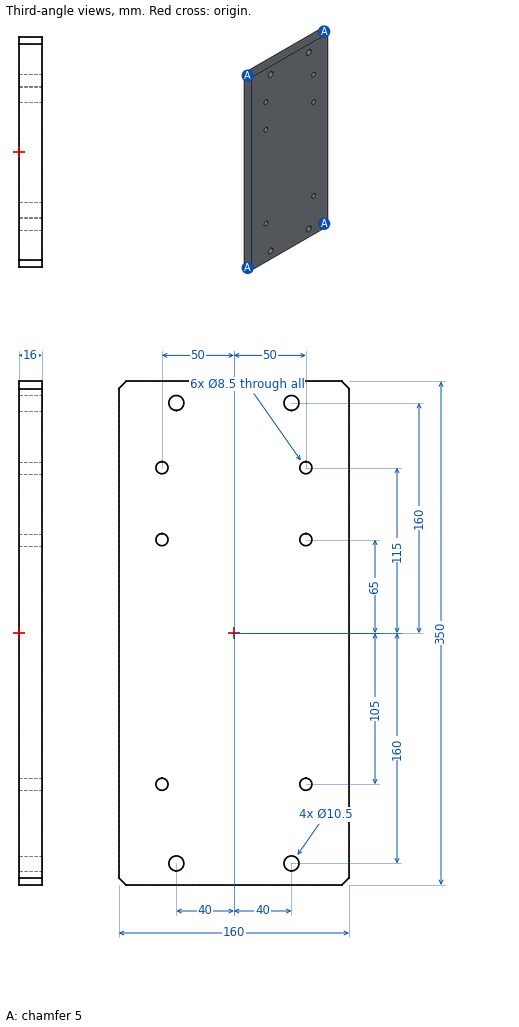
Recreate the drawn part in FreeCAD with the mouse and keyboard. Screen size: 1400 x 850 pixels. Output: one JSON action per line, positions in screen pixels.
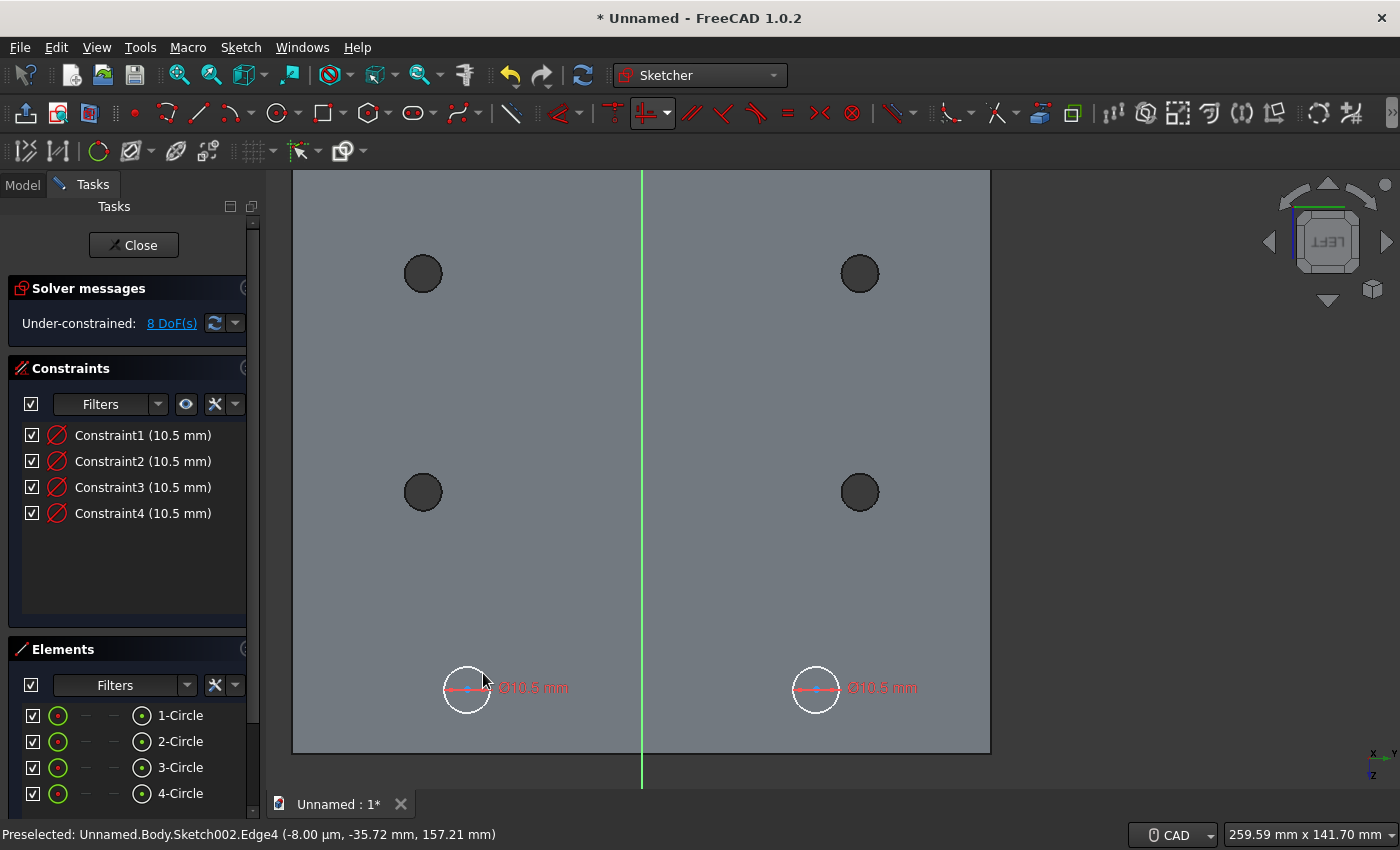
{"action": "scroll", "coordinate": [817, 691], "scroll_direction": "down", "scroll_amount": 6}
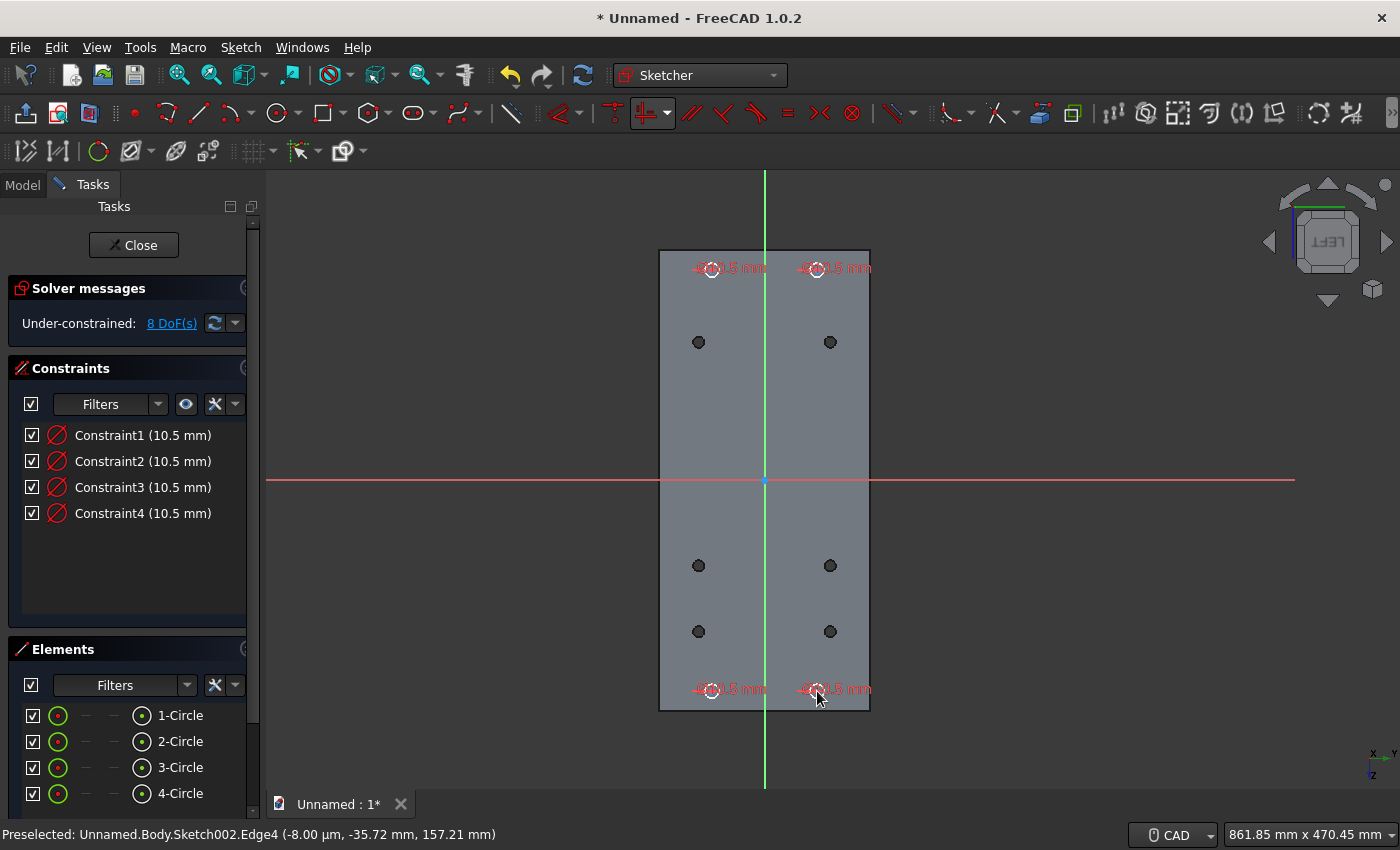
{"action": "left_click", "coordinate": [817, 270]}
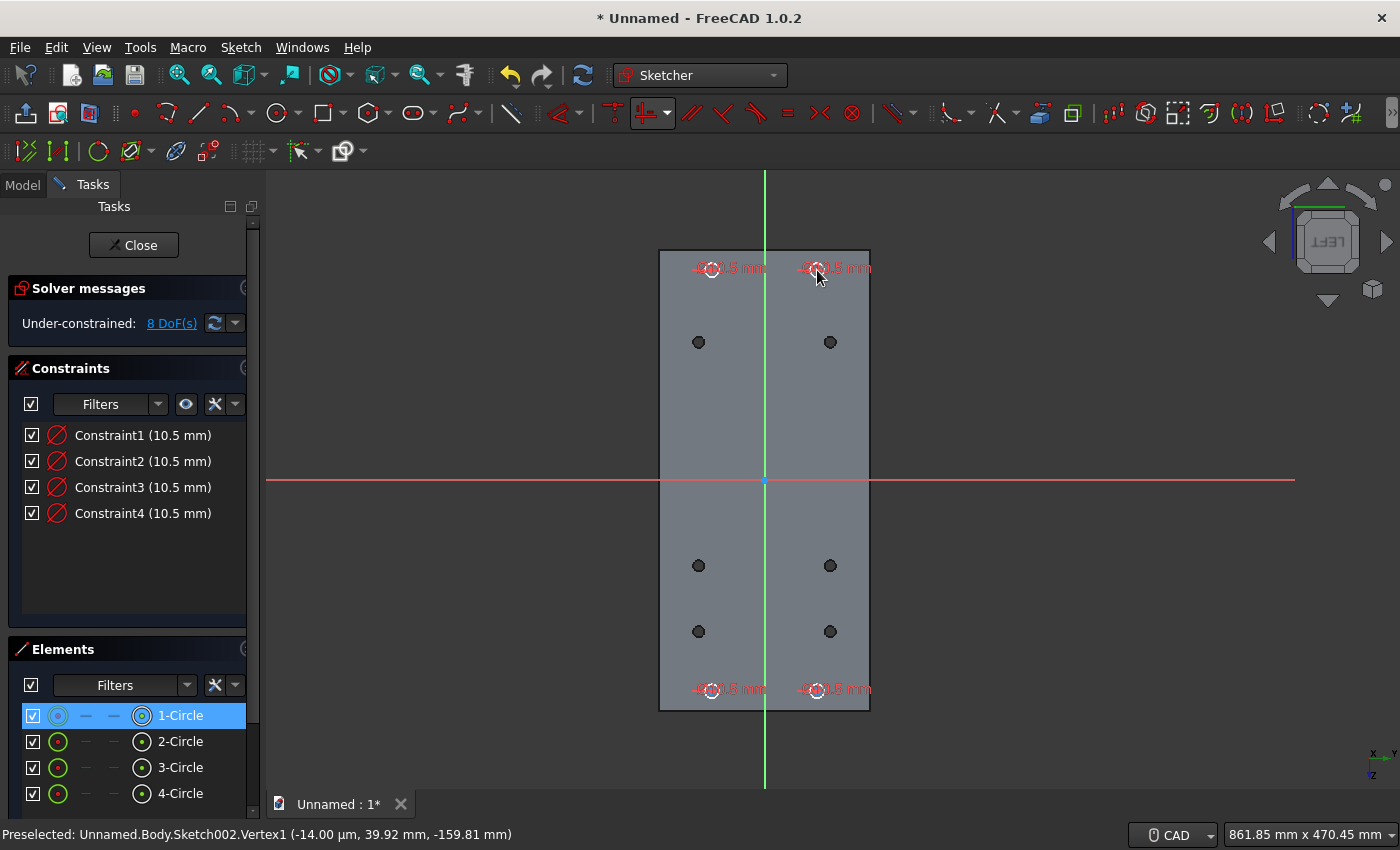
{"action": "left_click", "coordinate": [712, 270]}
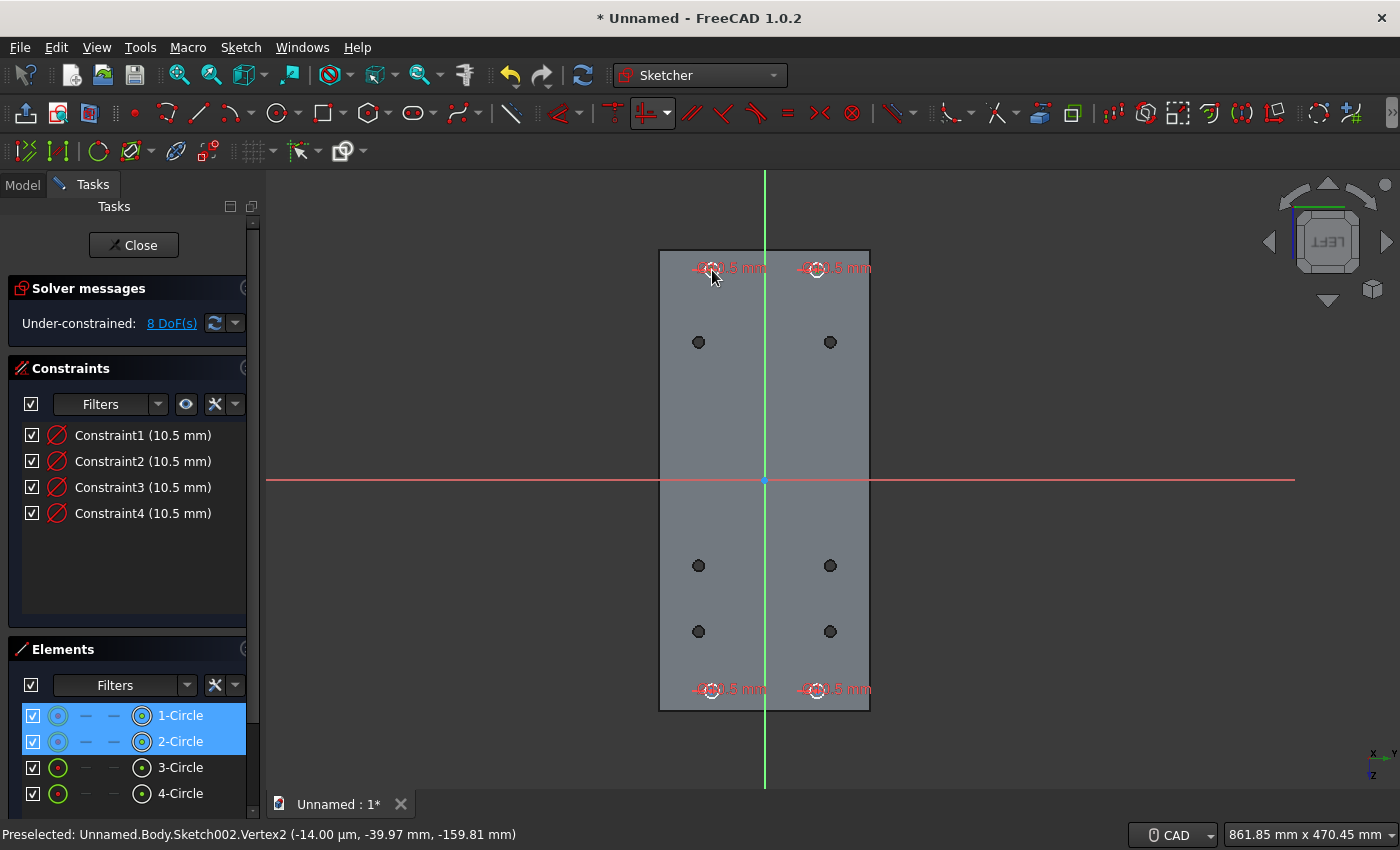
{"action": "key", "text": "h"}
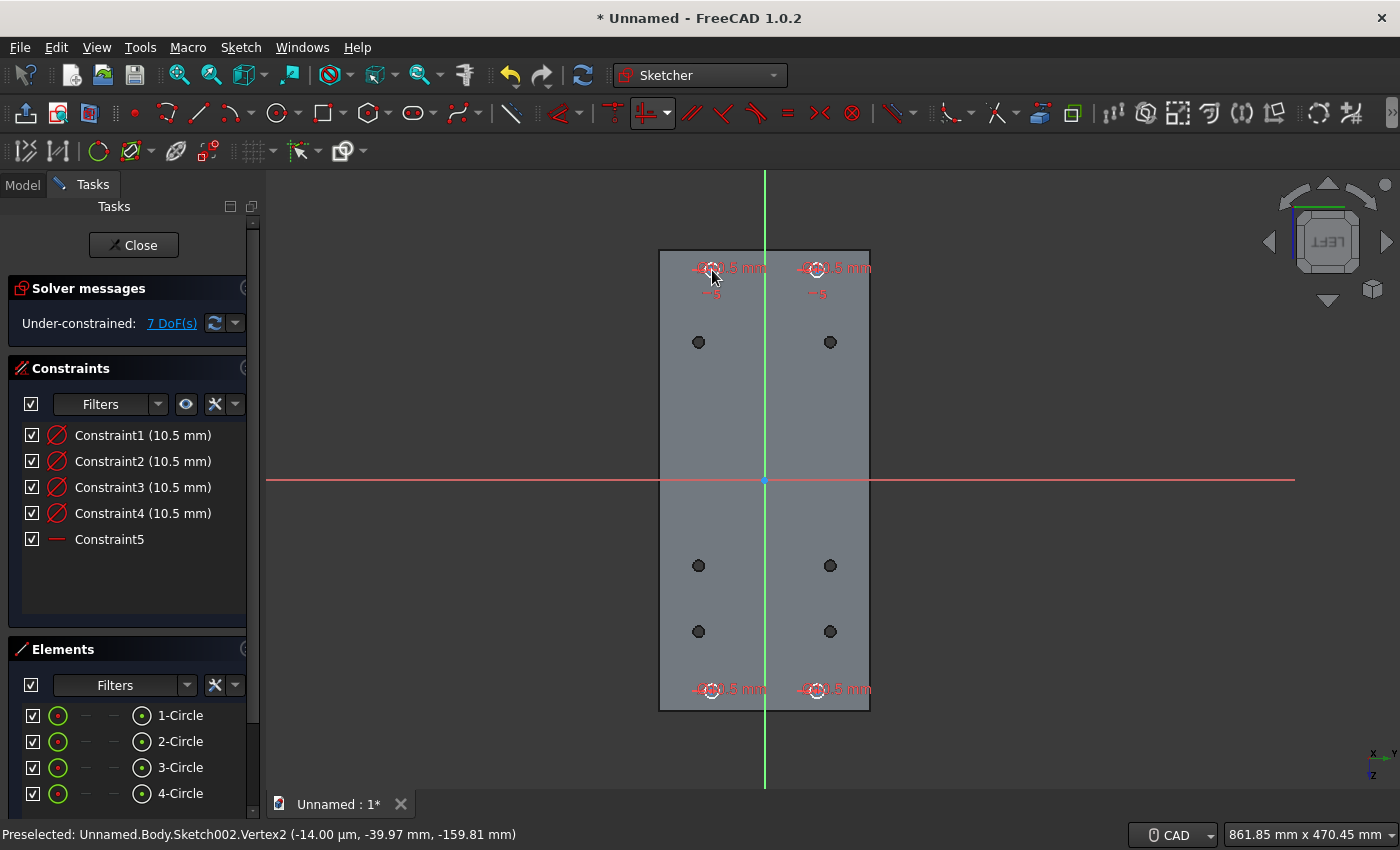
{"action": "left_click", "coordinate": [817, 270]}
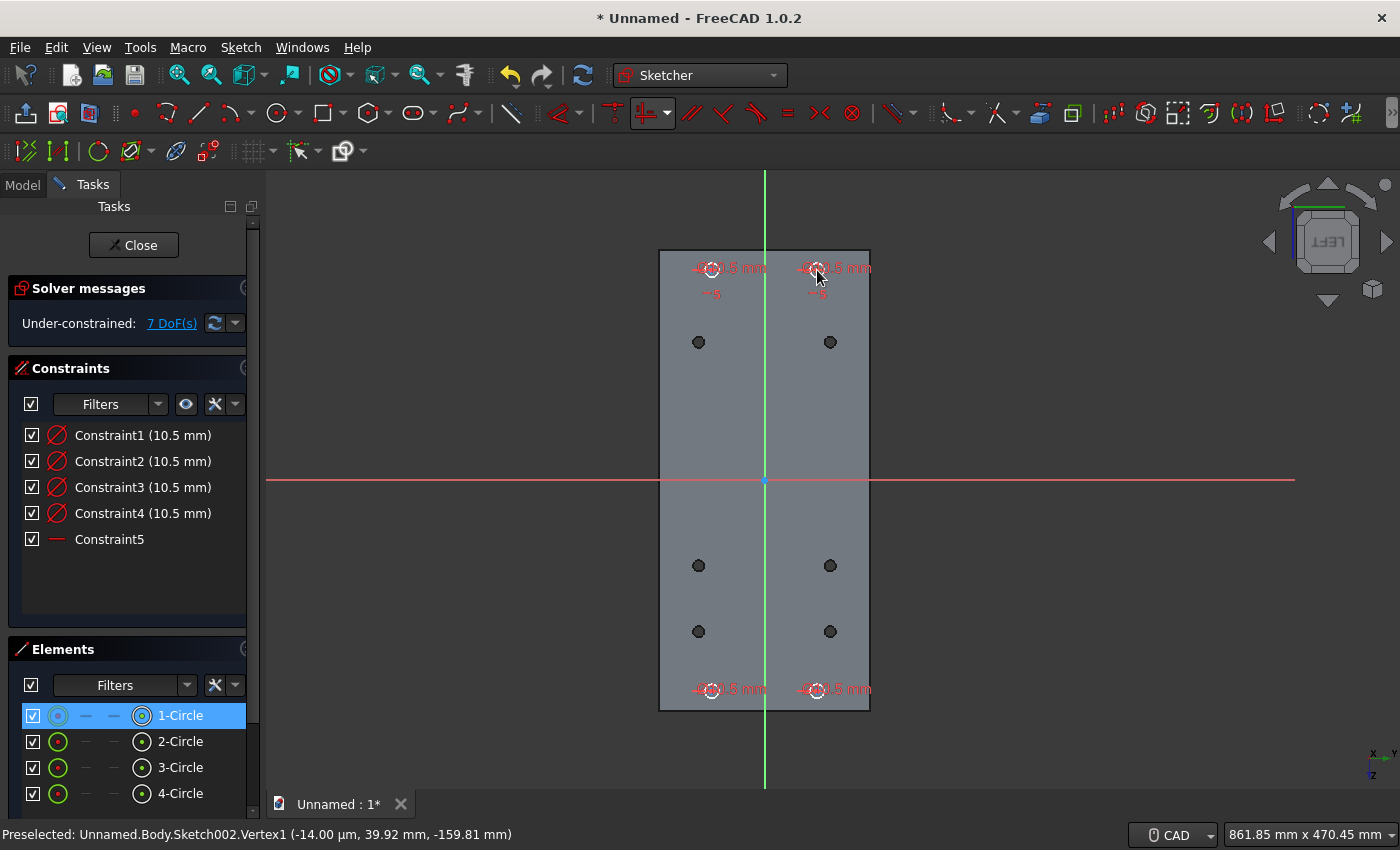
{"action": "left_click", "coordinate": [817, 691]}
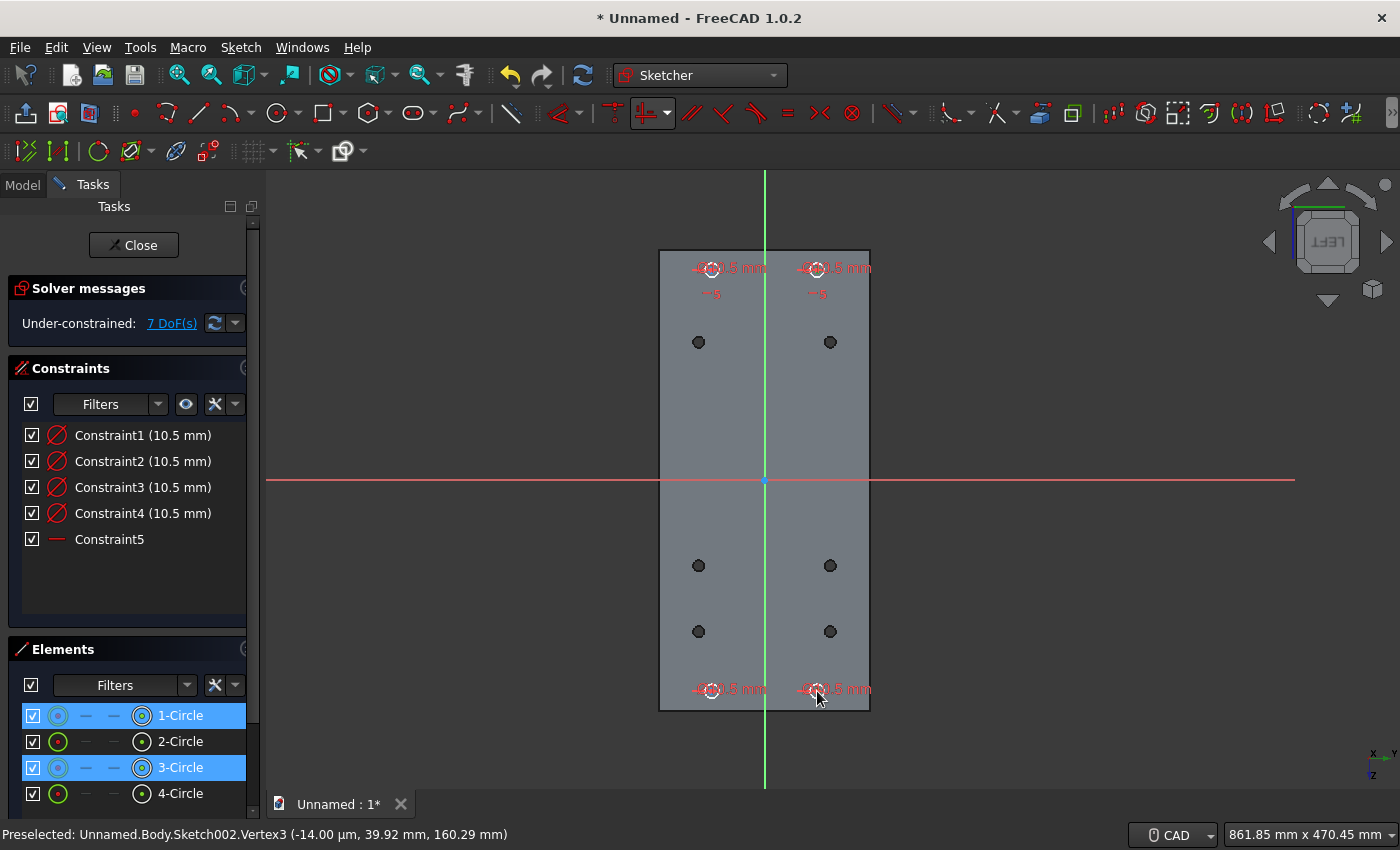
{"action": "key", "text": "v"}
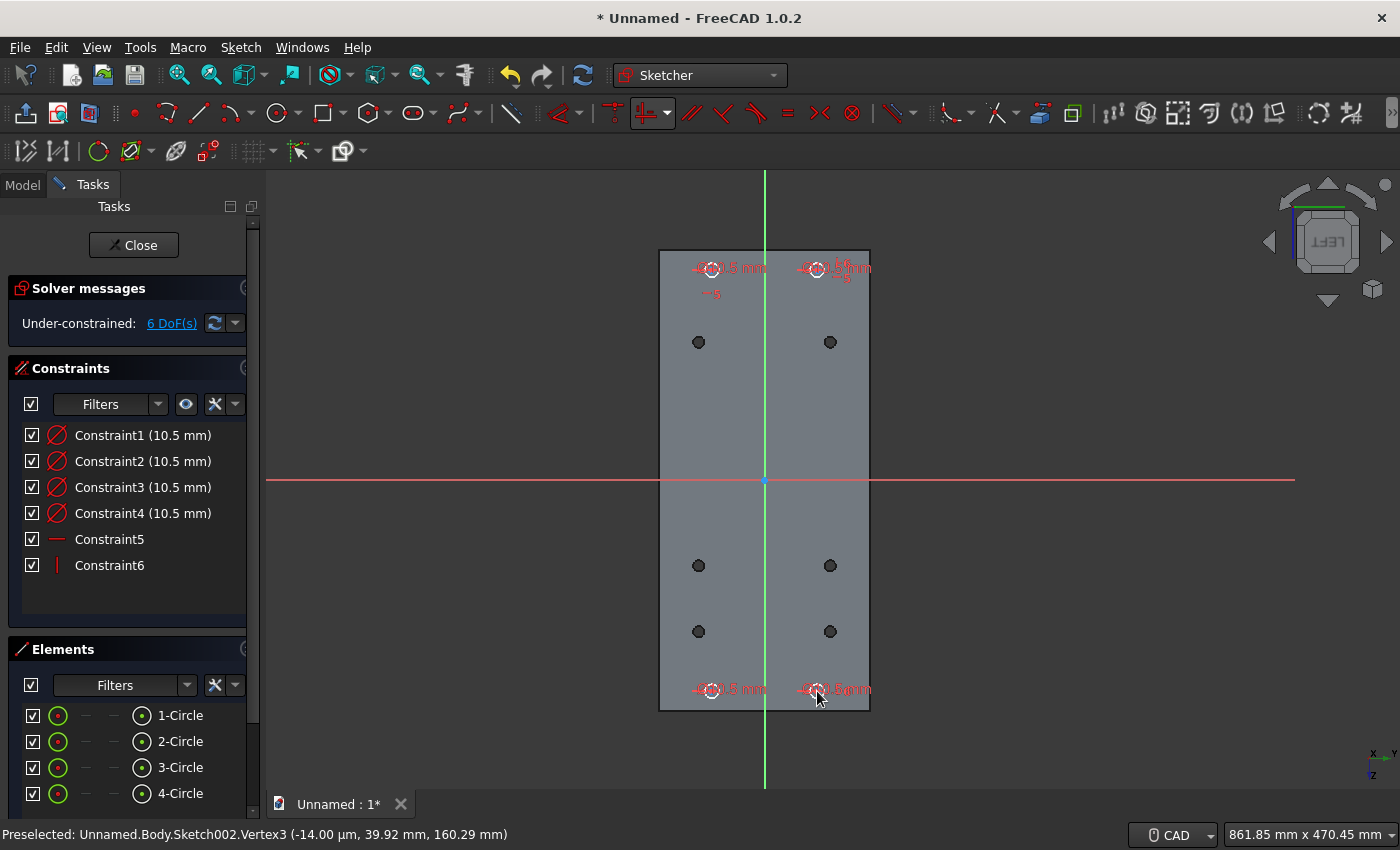
{"action": "left_click", "coordinate": [712, 270]}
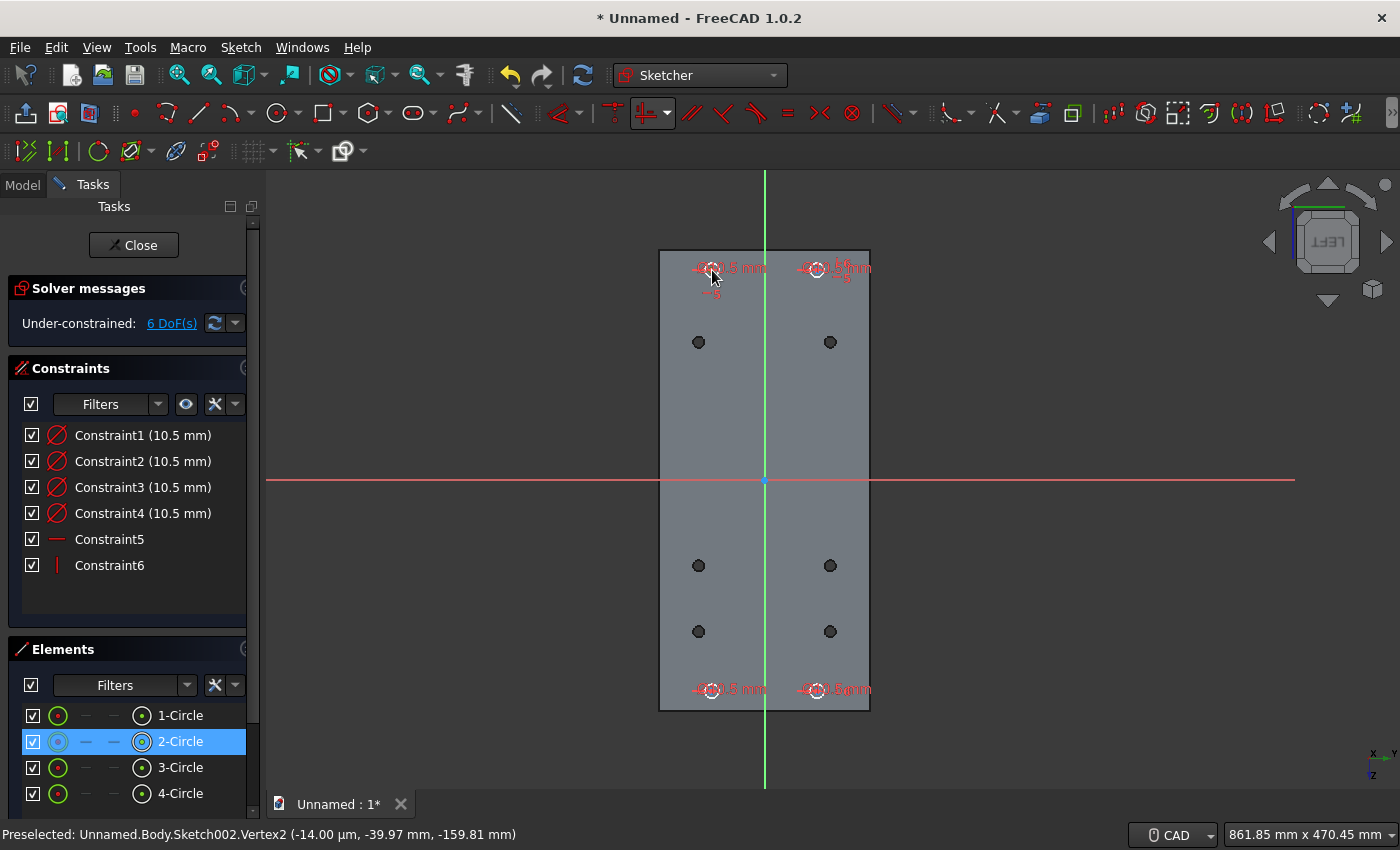
{"action": "left_click", "coordinate": [712, 691]}